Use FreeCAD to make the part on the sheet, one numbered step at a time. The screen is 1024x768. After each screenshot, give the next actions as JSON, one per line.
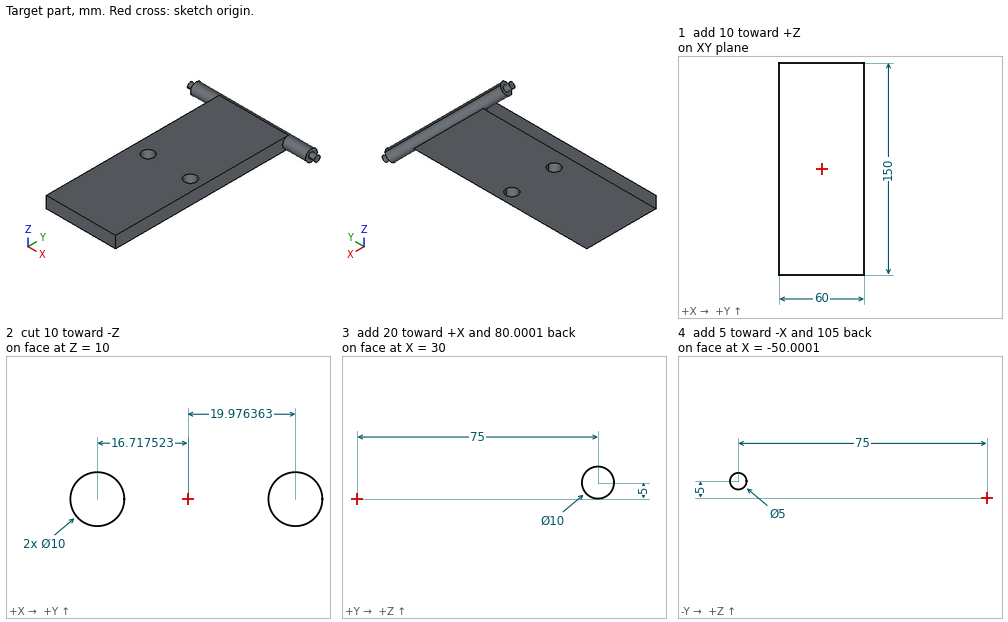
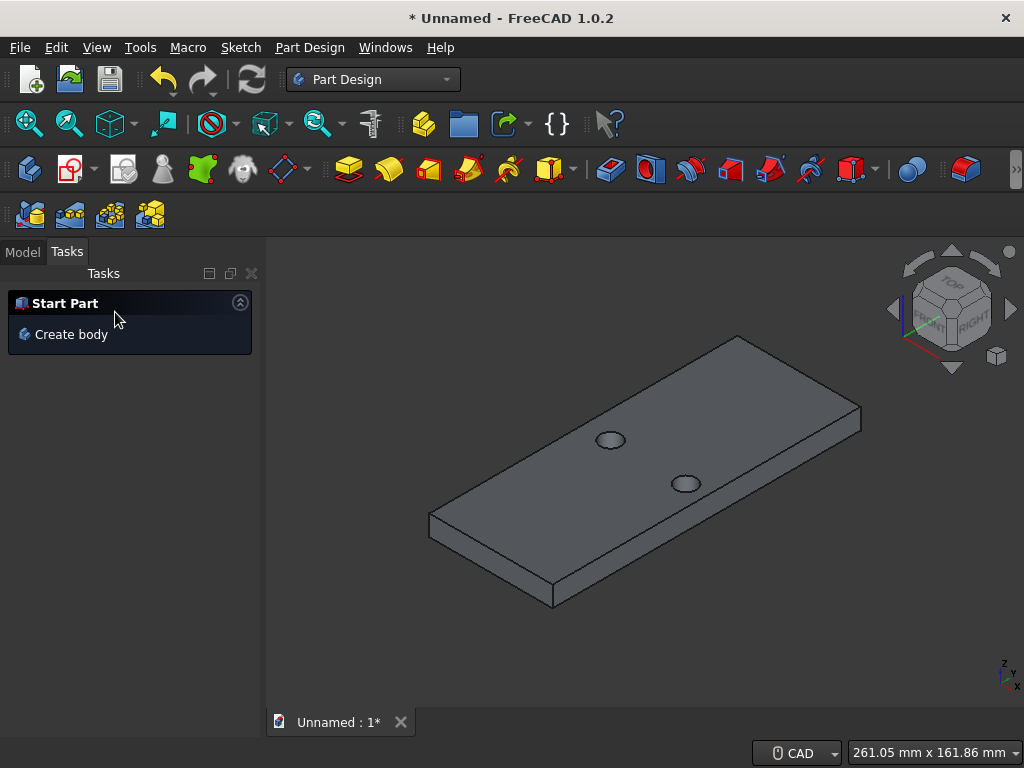
{"action": "left_click", "coordinate": [839, 430]}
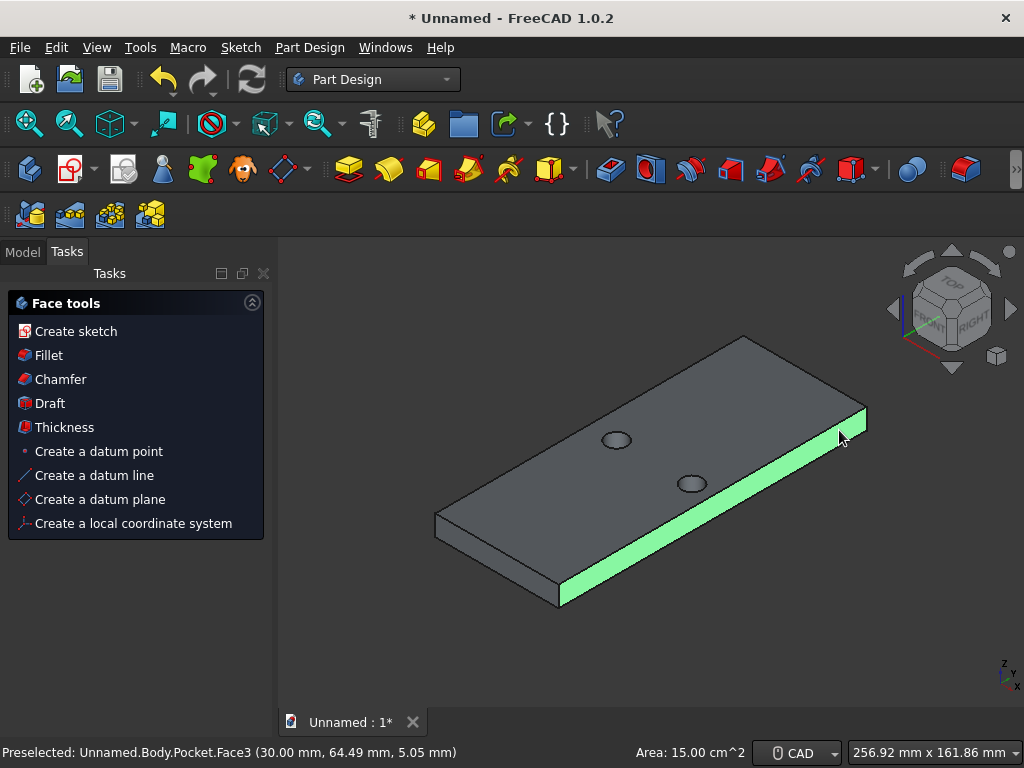
{"action": "left_click", "coordinate": [70, 170]}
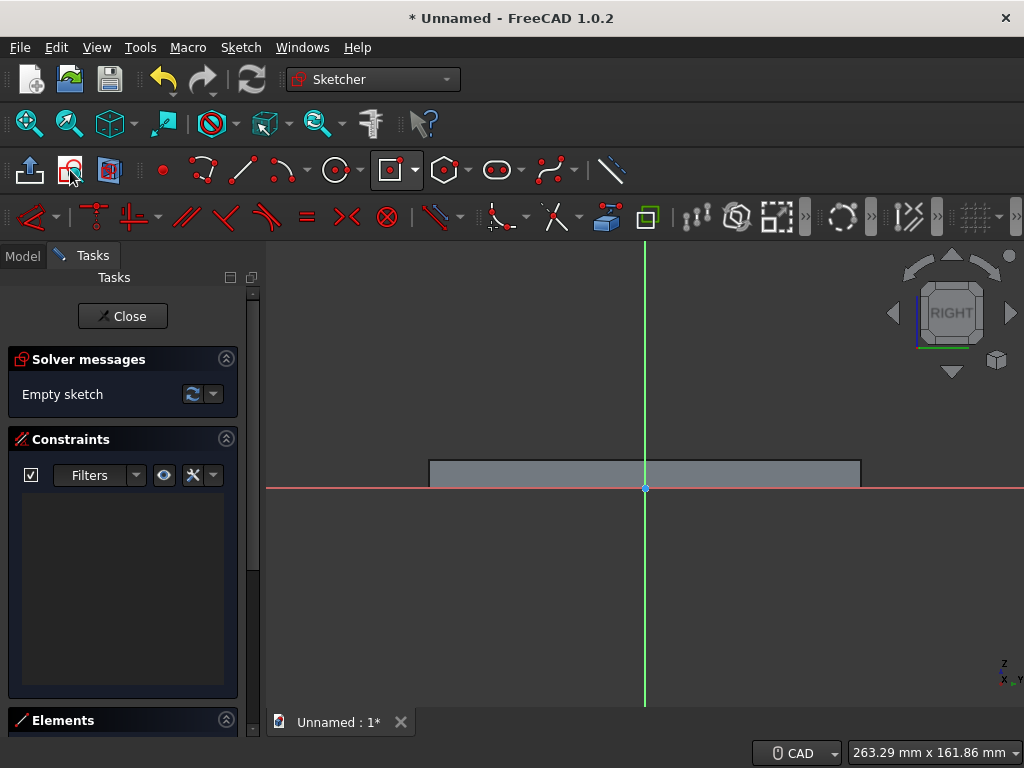
{"action": "scroll", "coordinate": [576, 474], "scroll_direction": "down", "scroll_amount": 5}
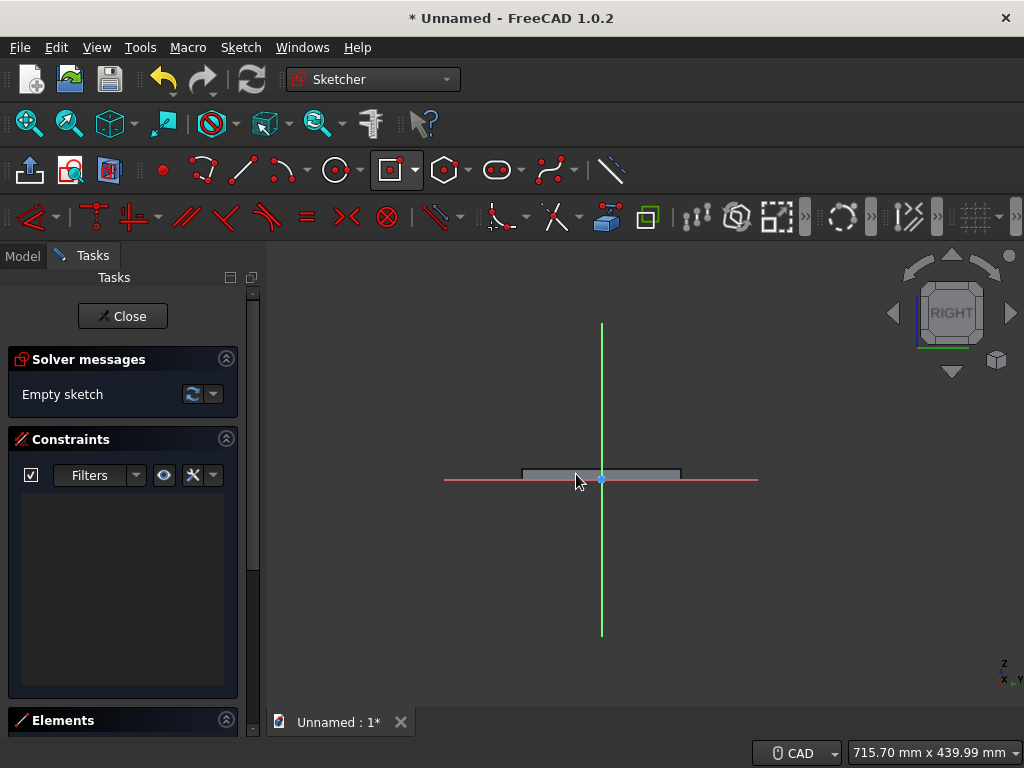
{"action": "scroll", "coordinate": [687, 474], "scroll_direction": "up", "scroll_amount": 15}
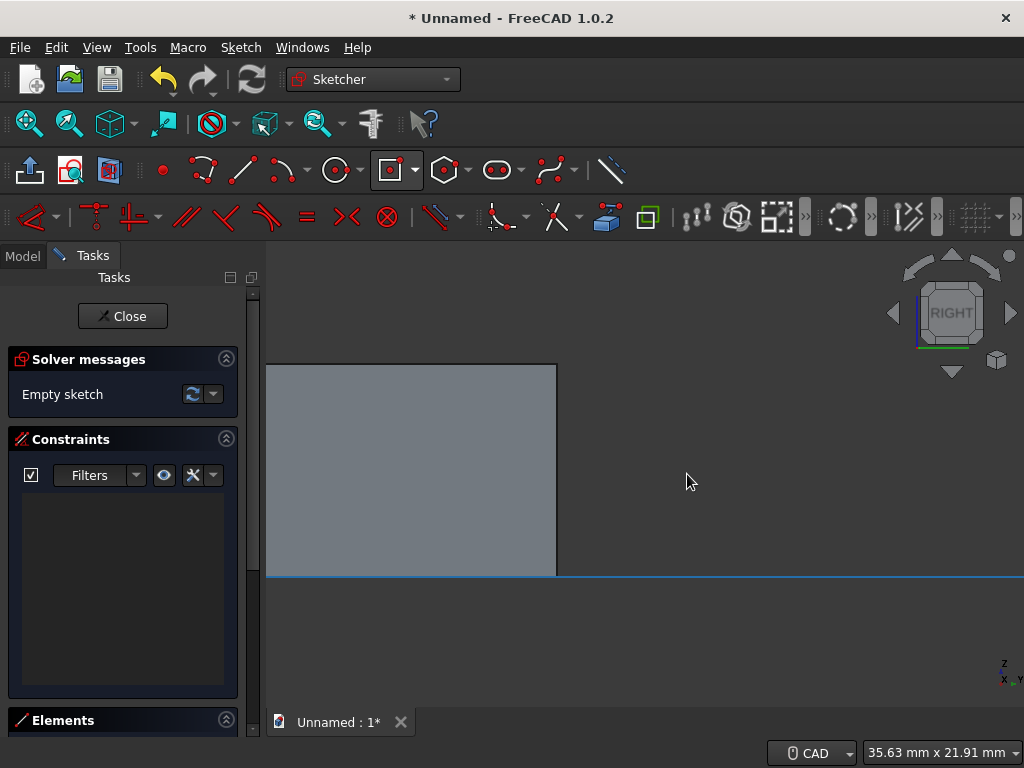
{"action": "scroll", "coordinate": [519, 464], "scroll_direction": "up", "scroll_amount": 2}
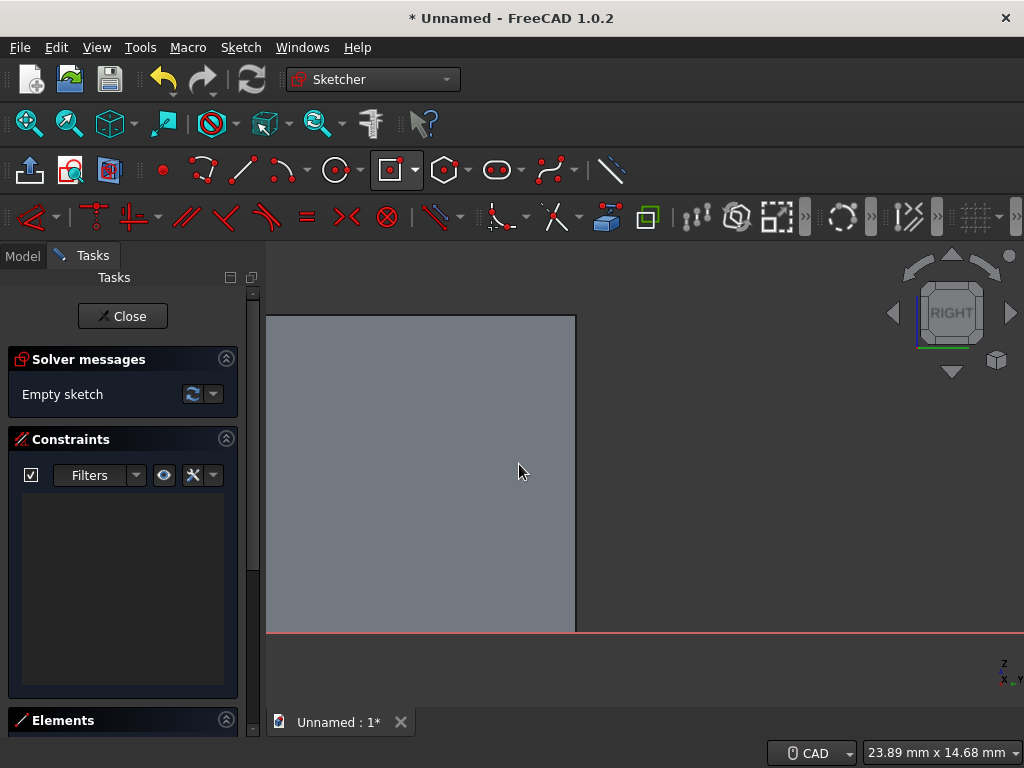
{"action": "left_click", "coordinate": [336, 170]}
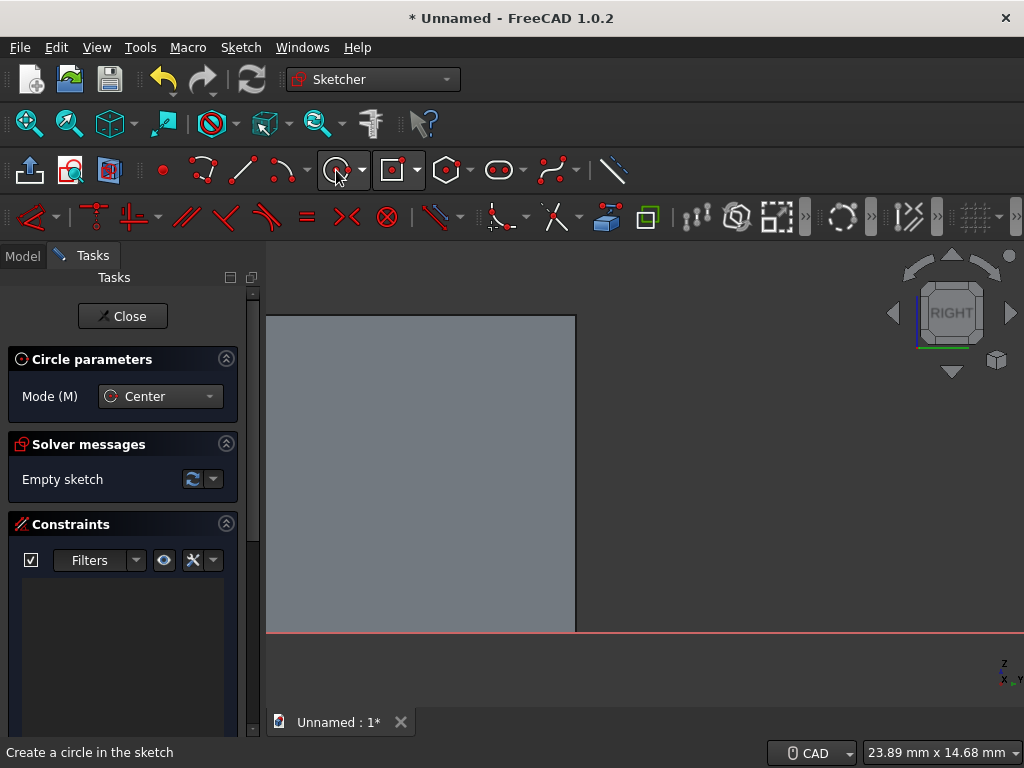
{"action": "left_click", "coordinate": [576, 474]}
{"action": "left_click", "coordinate": [688, 362]}
{"action": "key", "text": "Escape"}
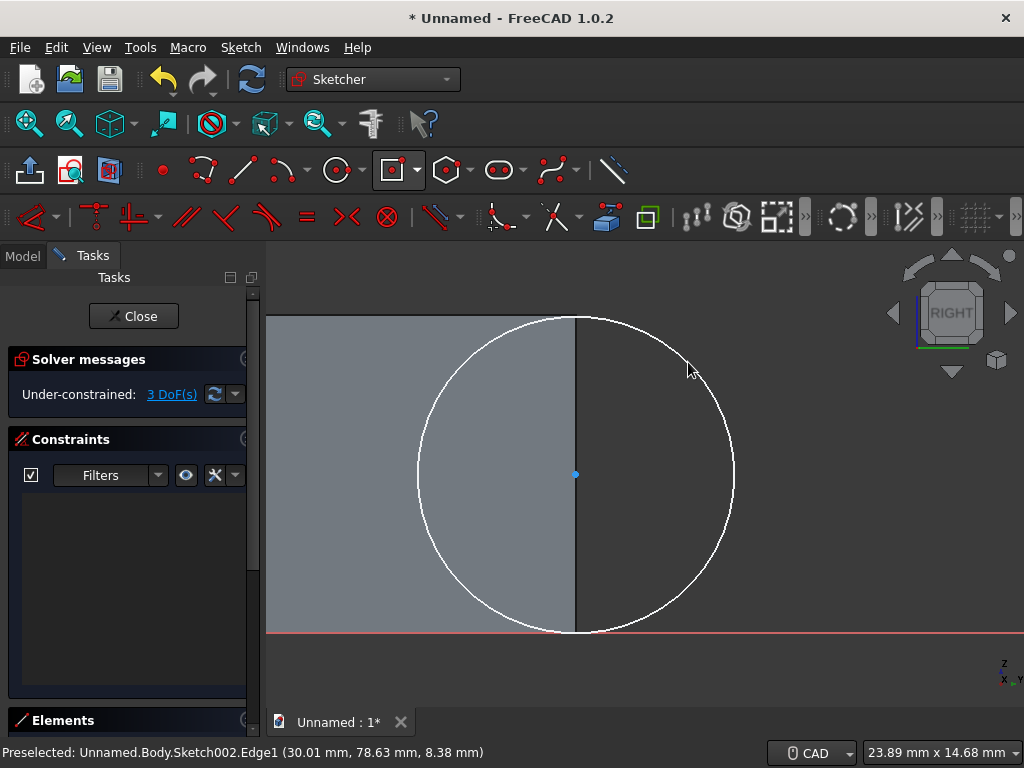
{"action": "left_click", "coordinate": [32, 218]}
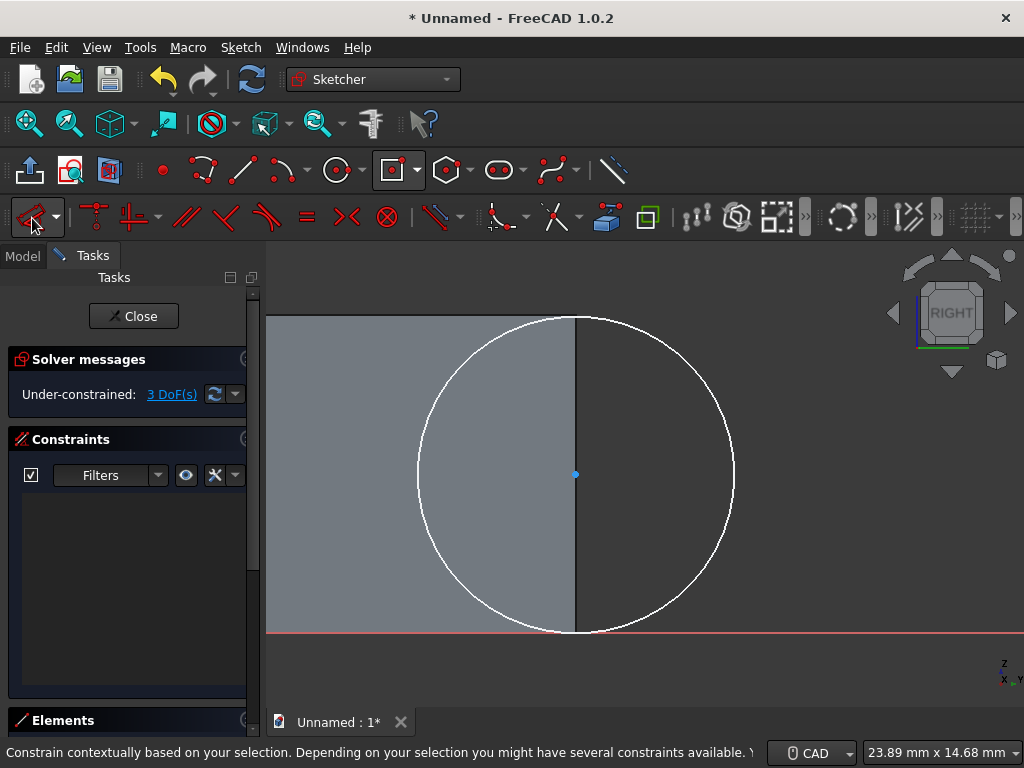
{"action": "left_click", "coordinate": [688, 363]}
{"action": "left_click", "coordinate": [711, 340]}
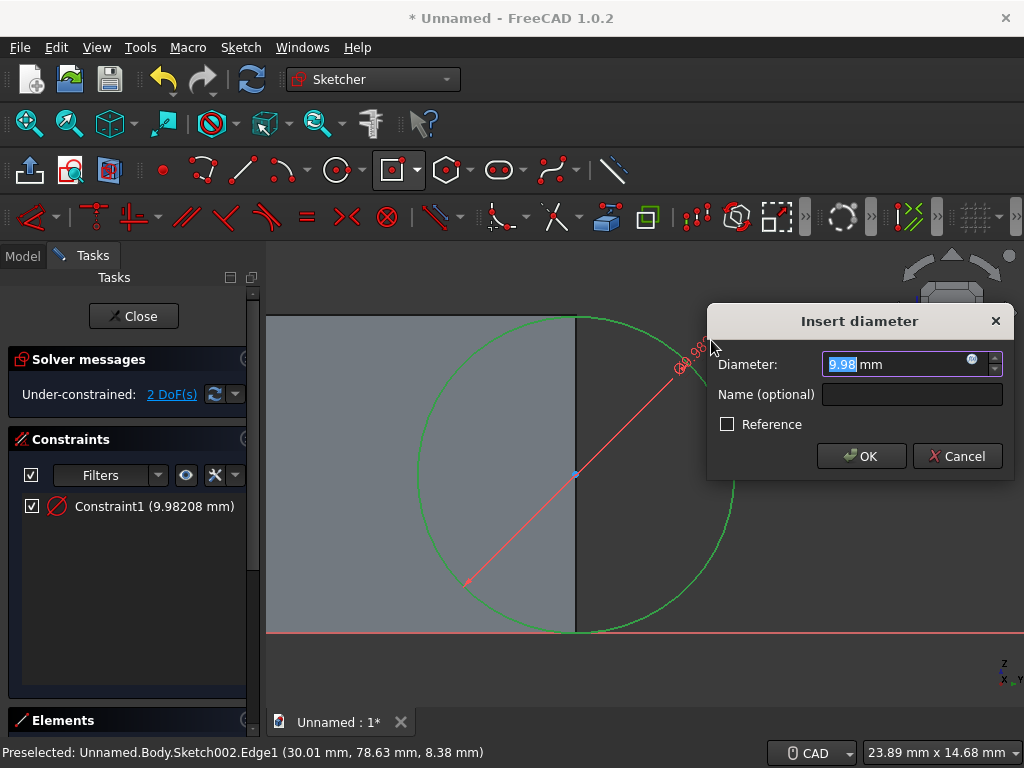
{"action": "type", "text": "10"}
{"action": "key", "text": "Return"}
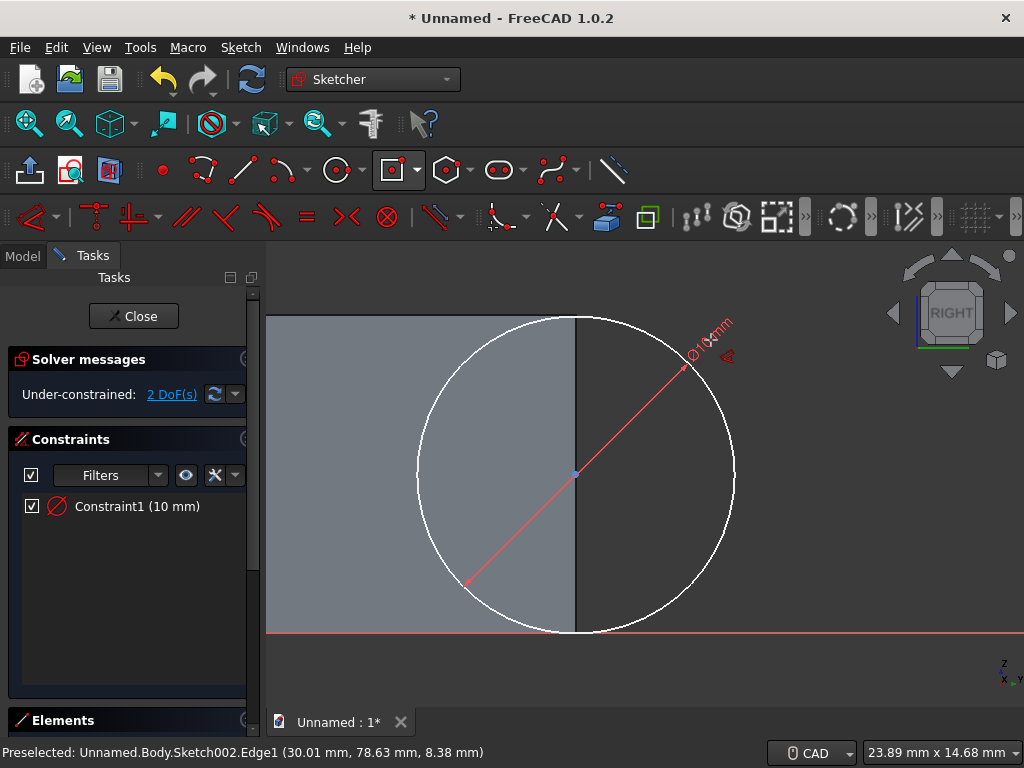
{"action": "left_click", "coordinate": [576, 475]}
{"action": "left_click", "coordinate": [610, 554]}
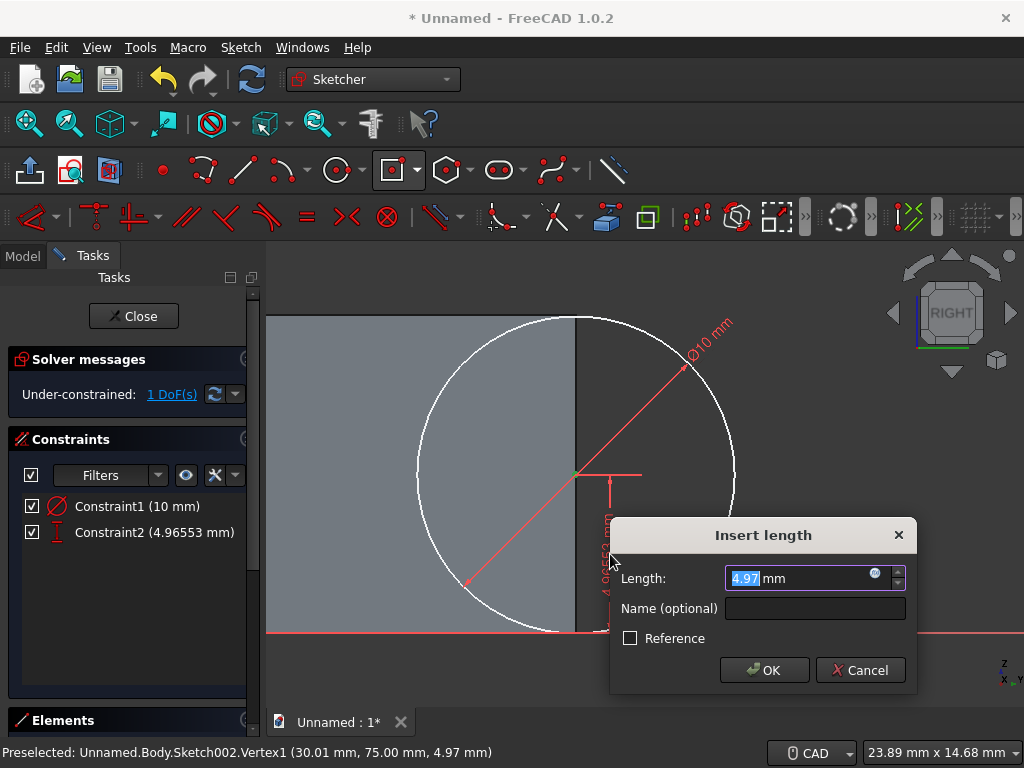
{"action": "type", "text": "5"}
{"action": "key", "text": "Return"}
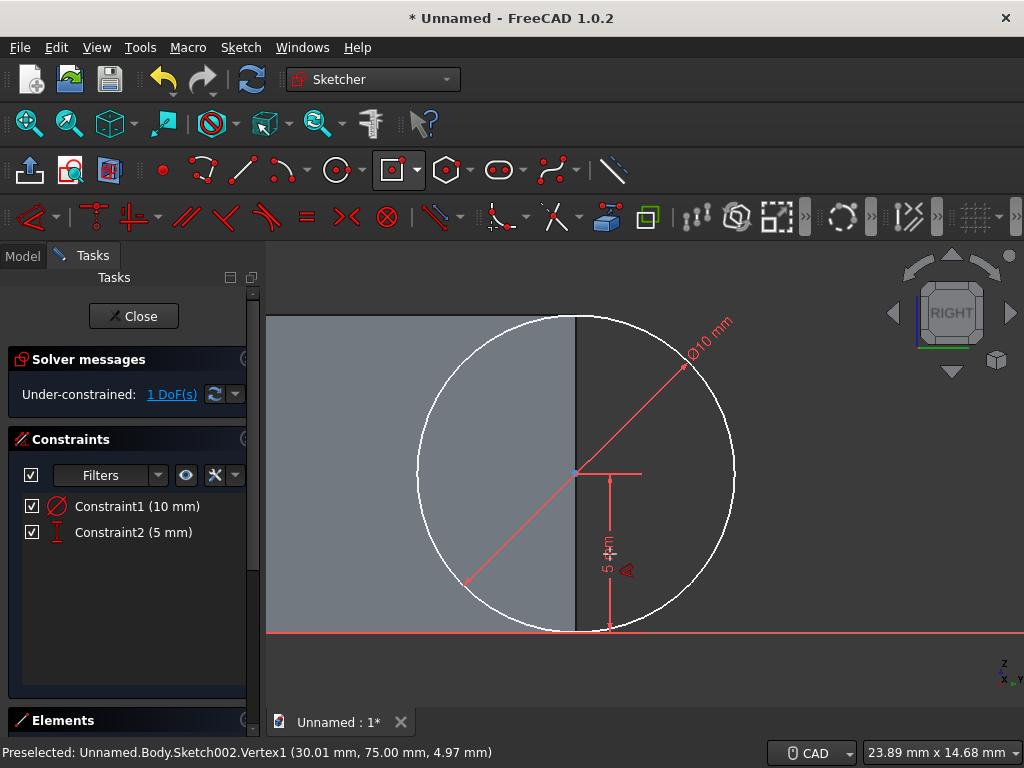
{"action": "left_click", "coordinate": [576, 474]}
{"action": "left_click", "coordinate": [435, 667]}